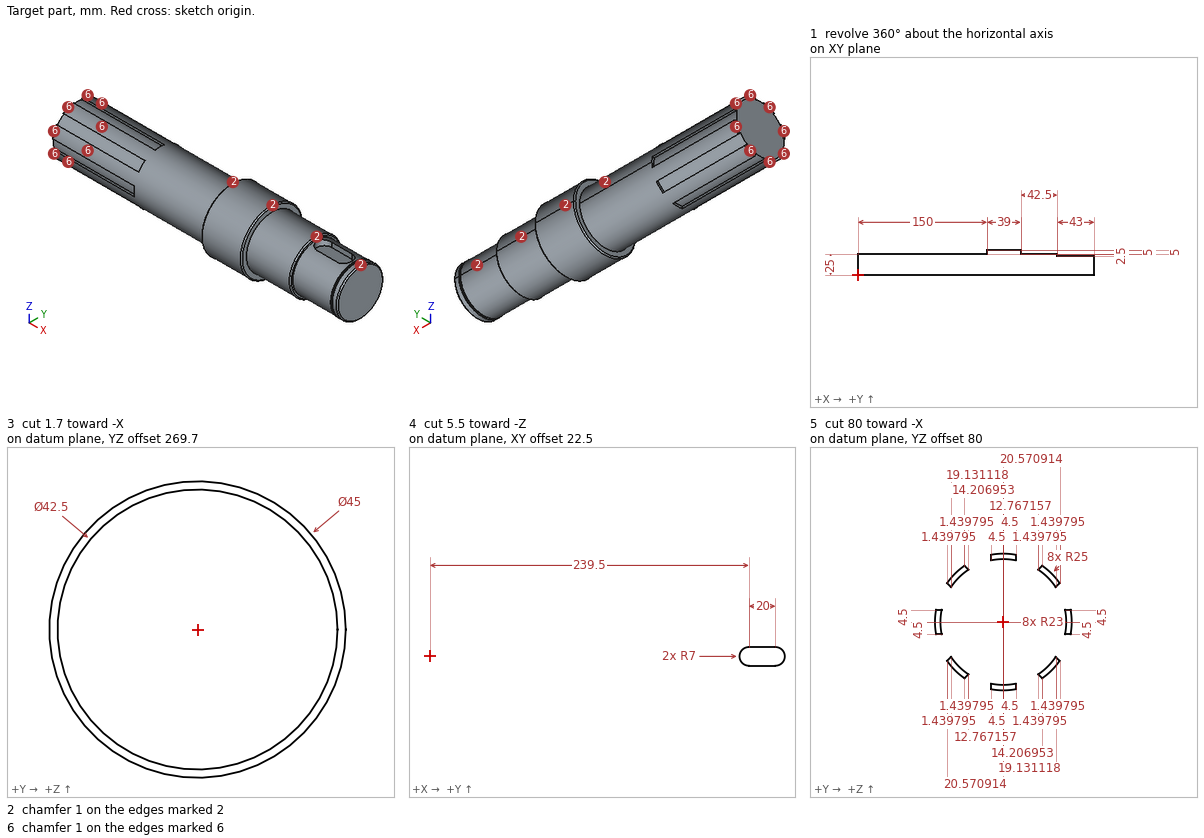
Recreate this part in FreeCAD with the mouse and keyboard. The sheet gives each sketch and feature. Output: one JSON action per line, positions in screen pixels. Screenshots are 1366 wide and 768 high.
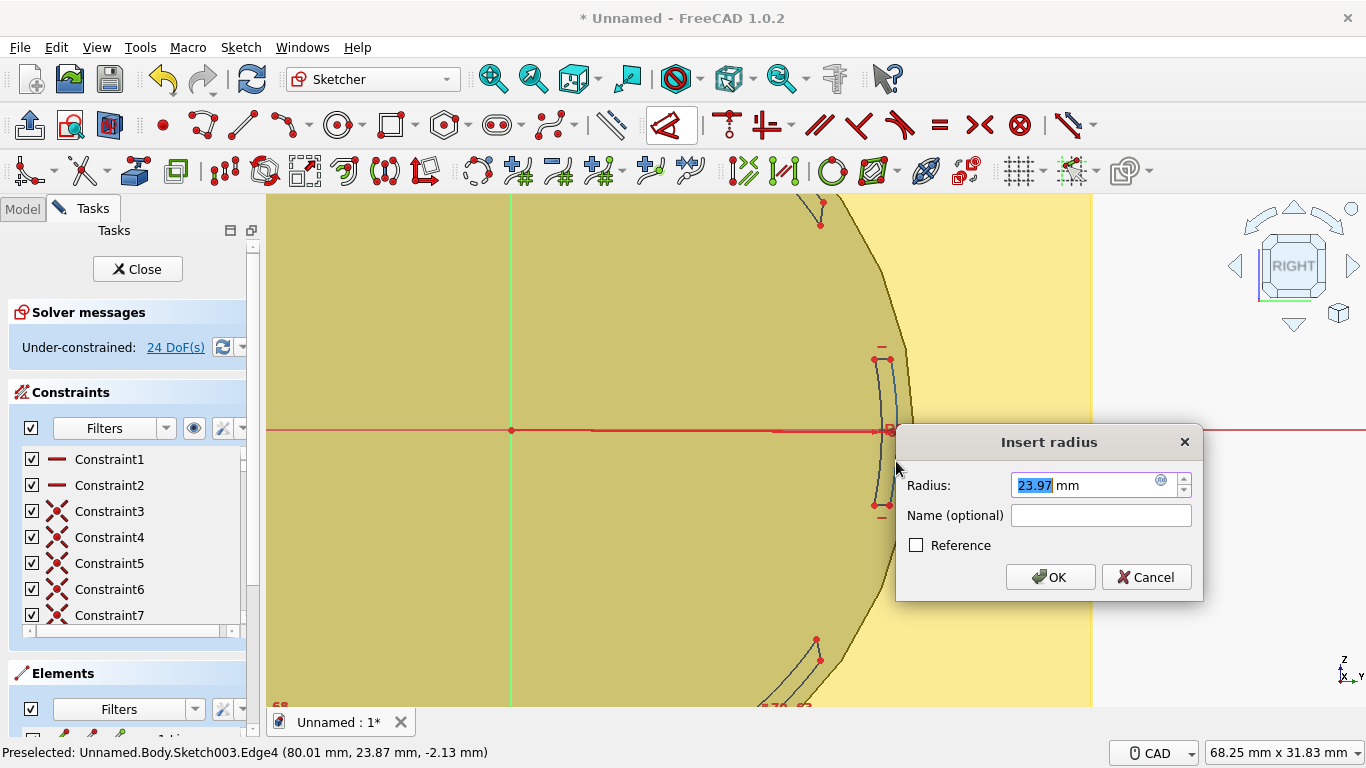
{"action": "type", "text": "25"}
{"action": "key", "text": "Return"}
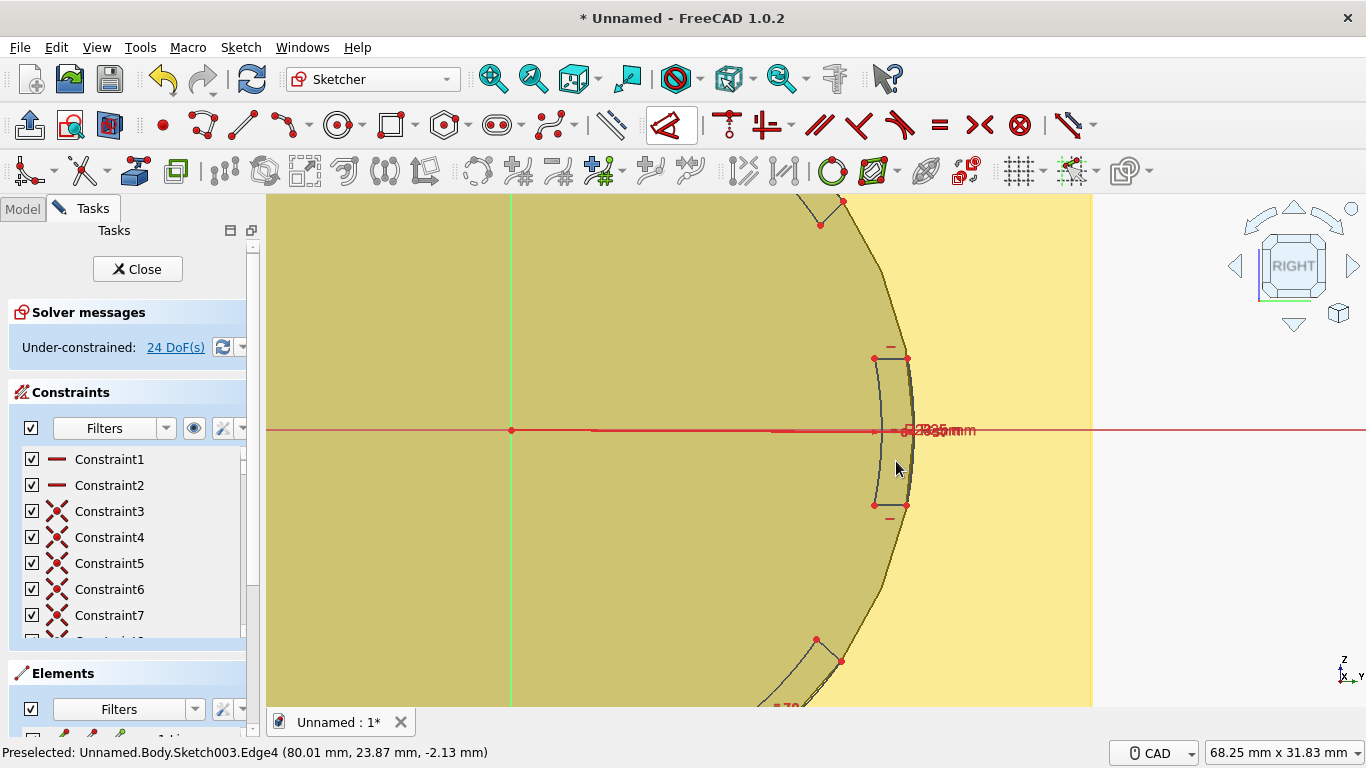
{"action": "left_click", "coordinate": [907, 505]}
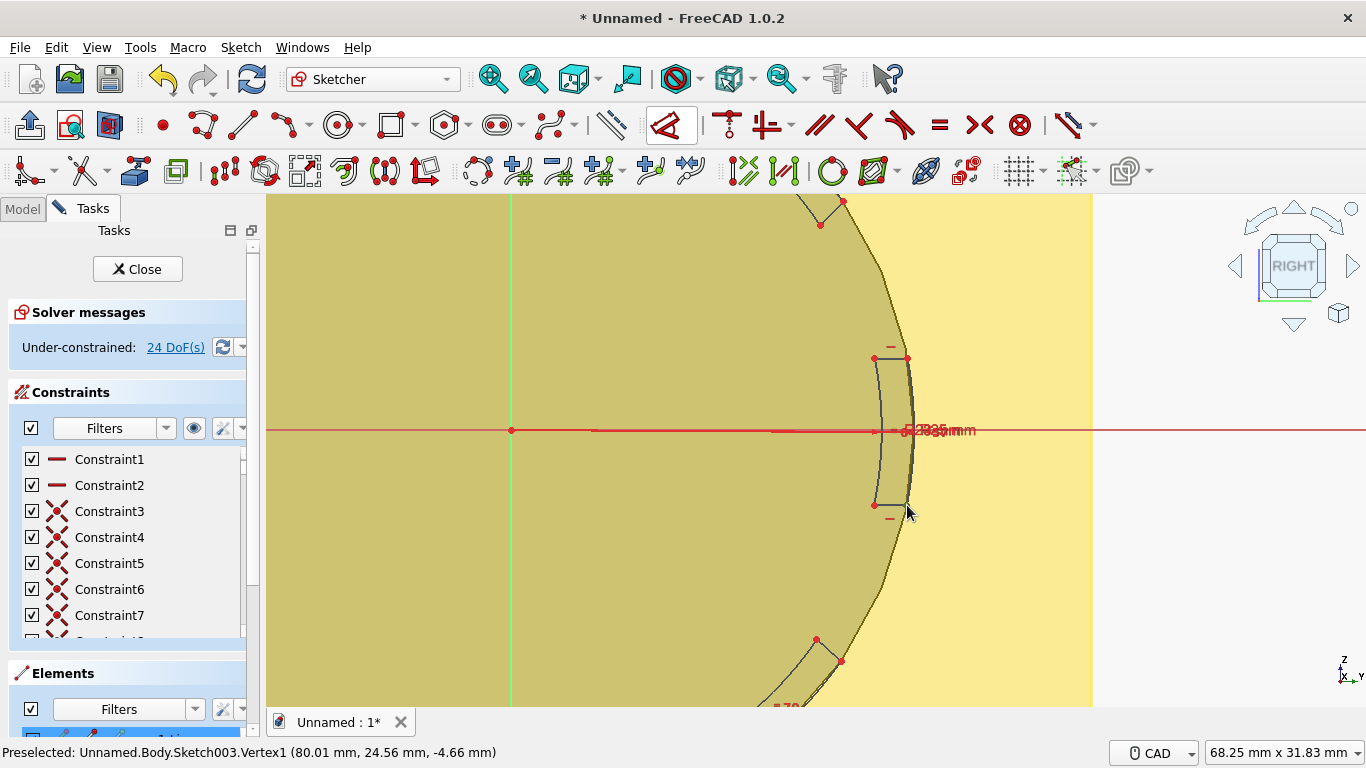
{"action": "key", "text": "i"}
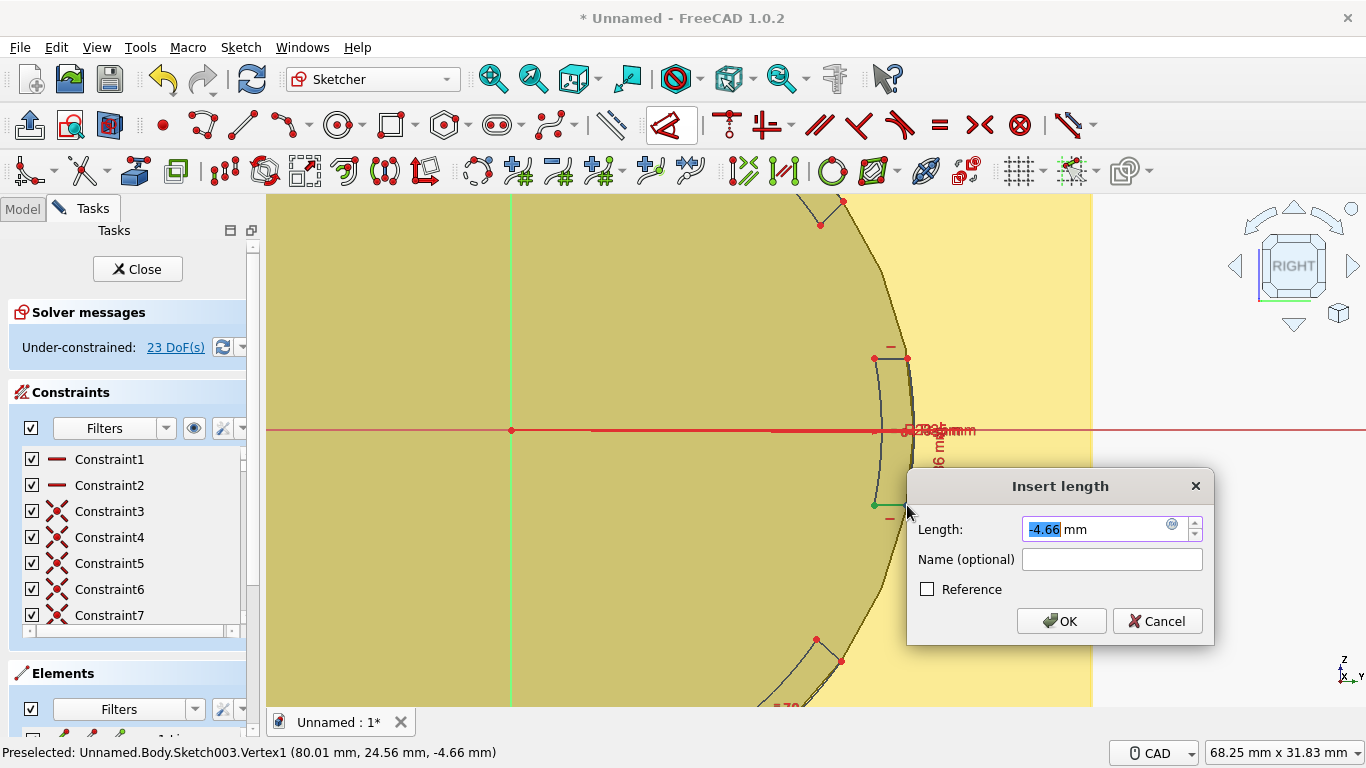
{"action": "type", "text": "-4.5"}
{"action": "key", "text": "Return"}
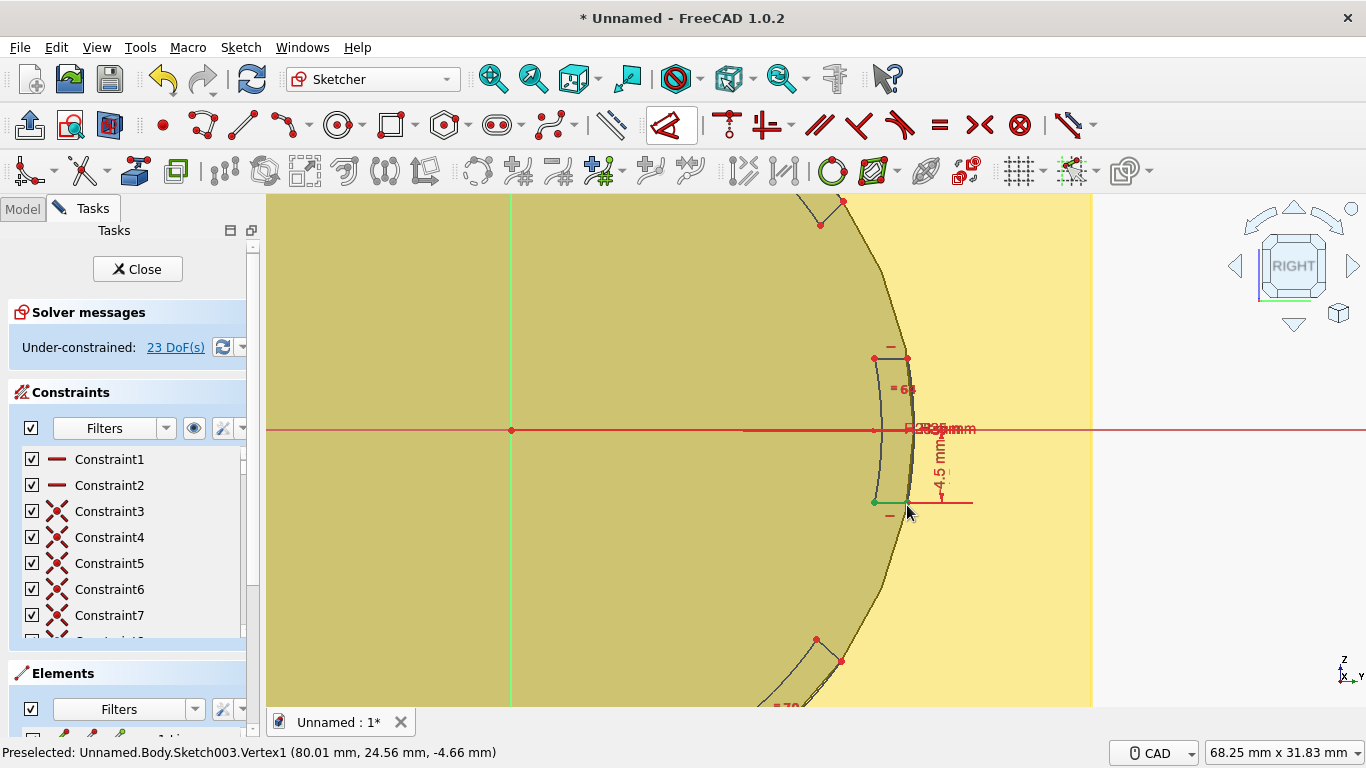
{"action": "left_click", "coordinate": [875, 359]}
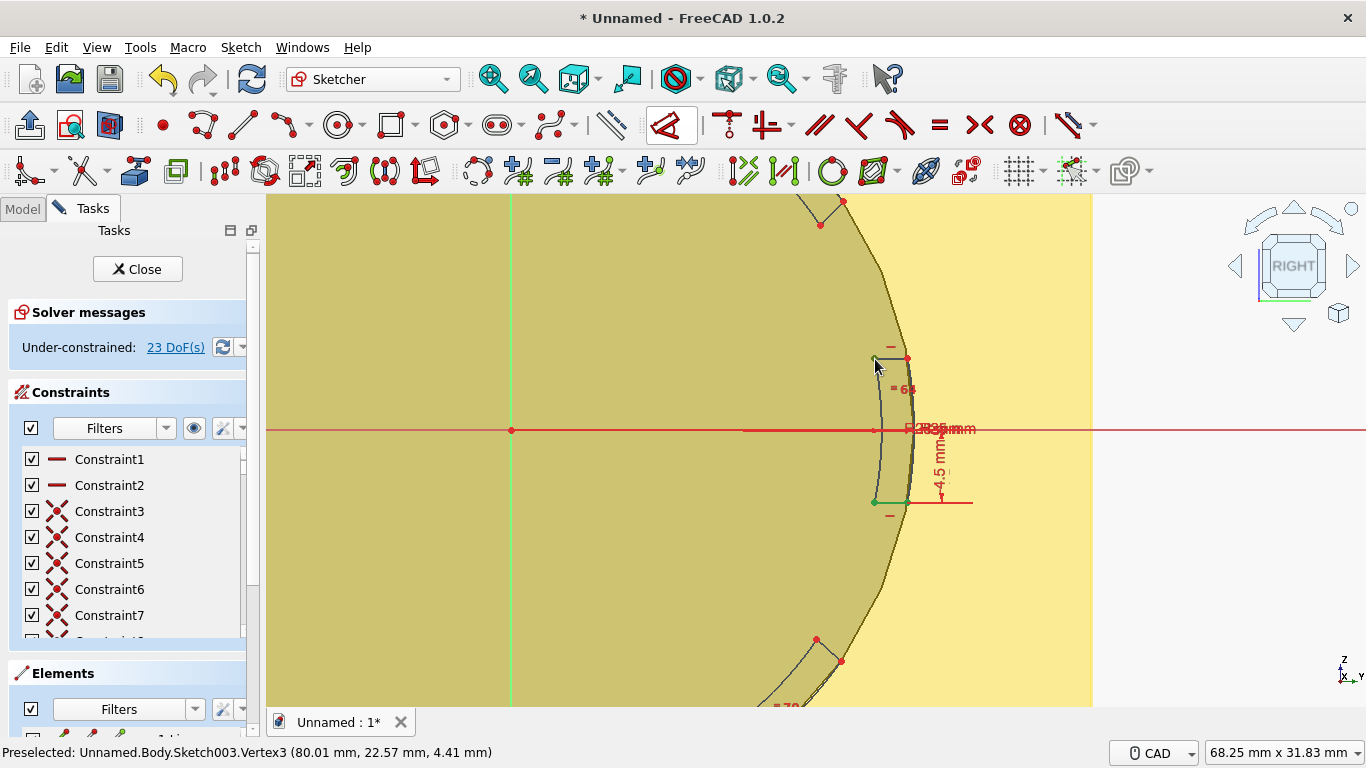
{"action": "left_click", "coordinate": [692, 126]}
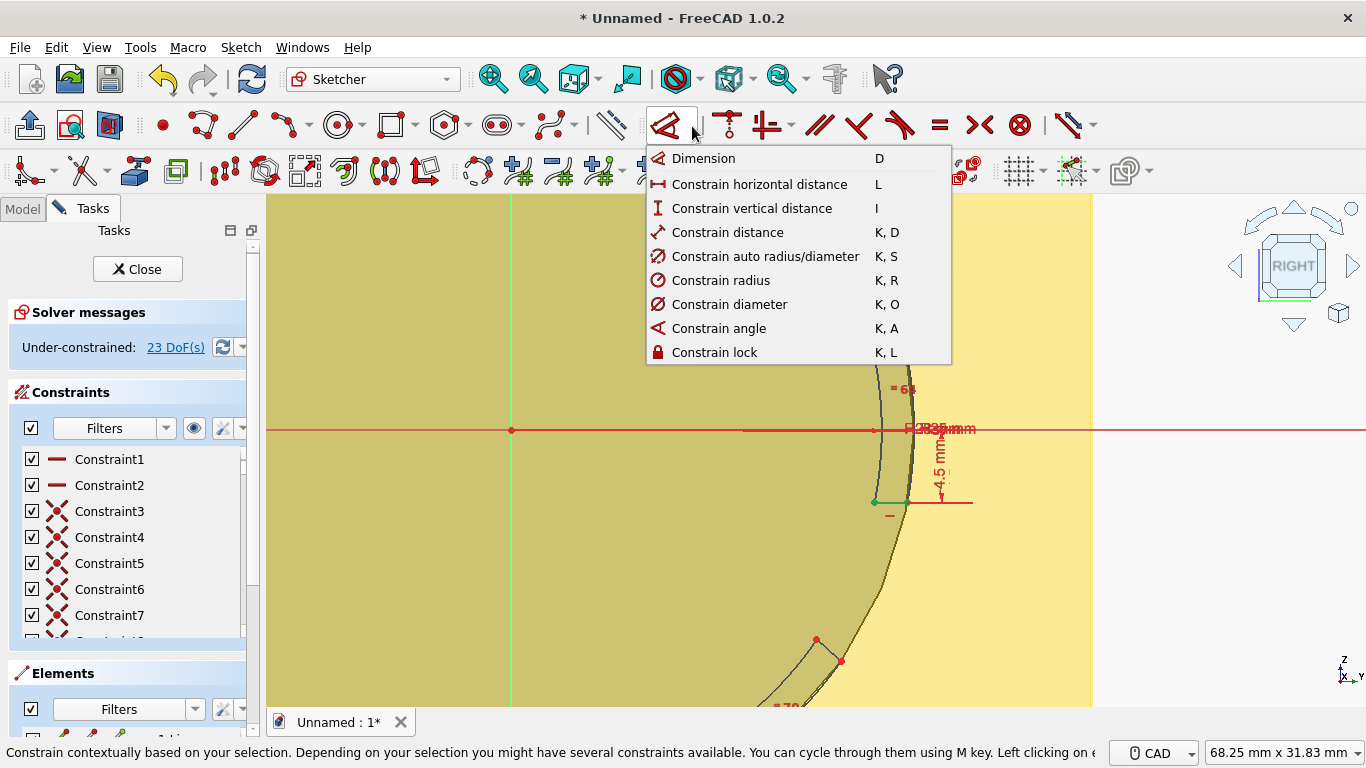
{"action": "left_click", "coordinate": [799, 208]}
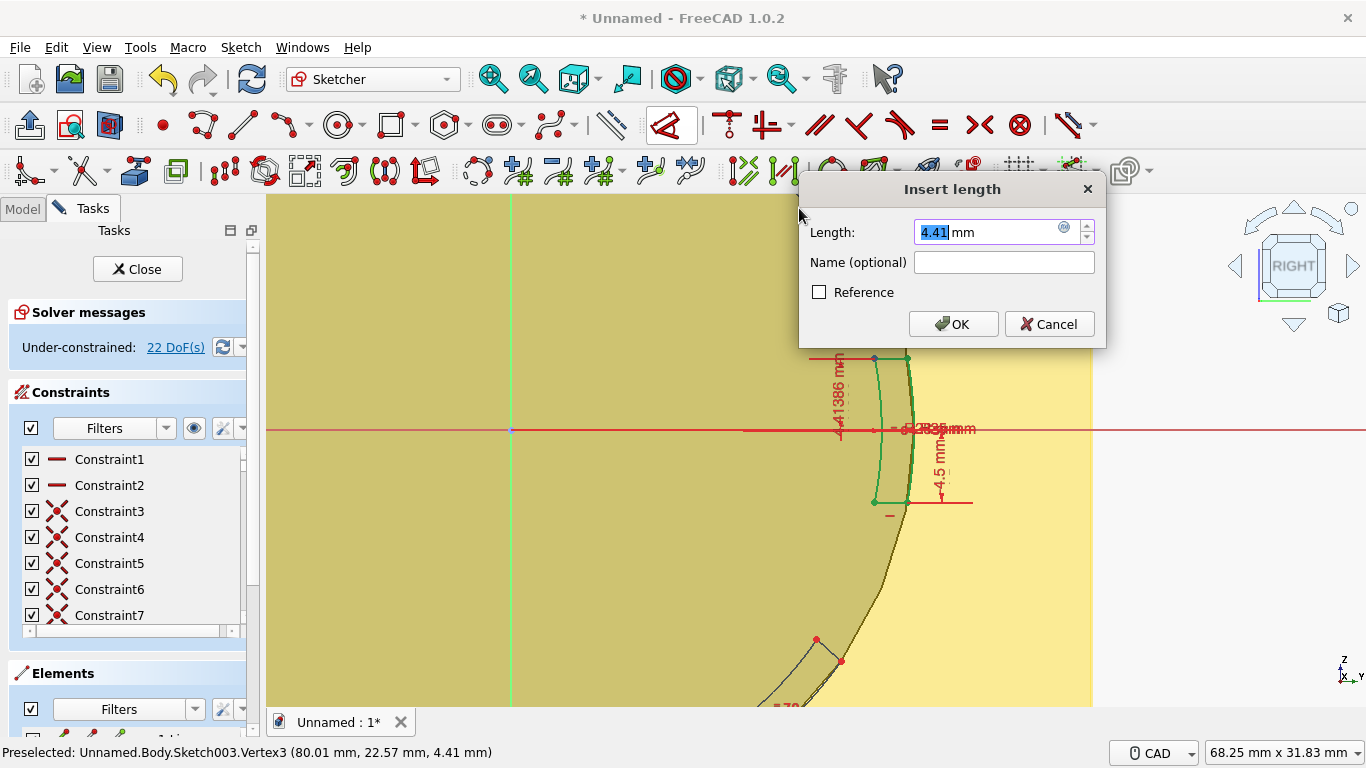
{"action": "type", "text": "4.5"}
{"action": "key", "text": "Return"}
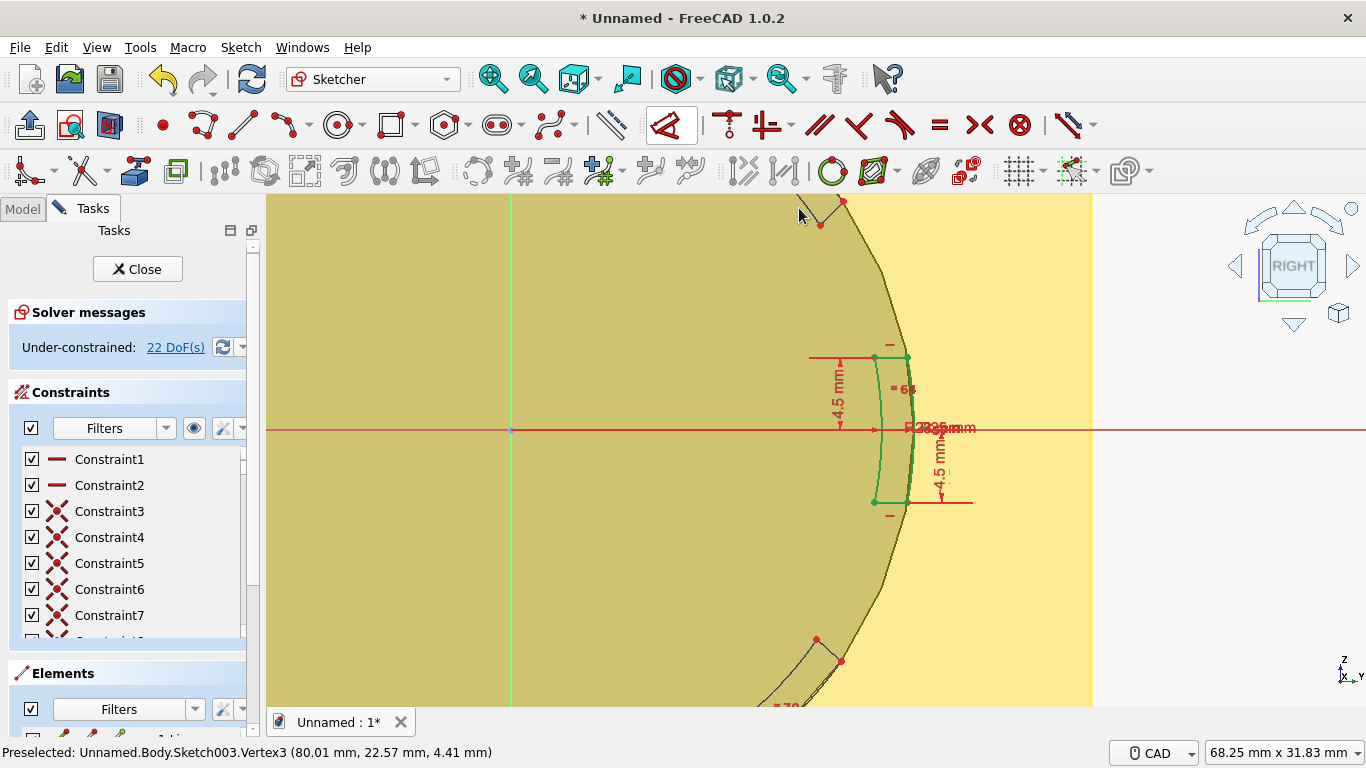
{"action": "scroll", "coordinate": [885, 462], "scroll_direction": "down", "scroll_amount": 5}